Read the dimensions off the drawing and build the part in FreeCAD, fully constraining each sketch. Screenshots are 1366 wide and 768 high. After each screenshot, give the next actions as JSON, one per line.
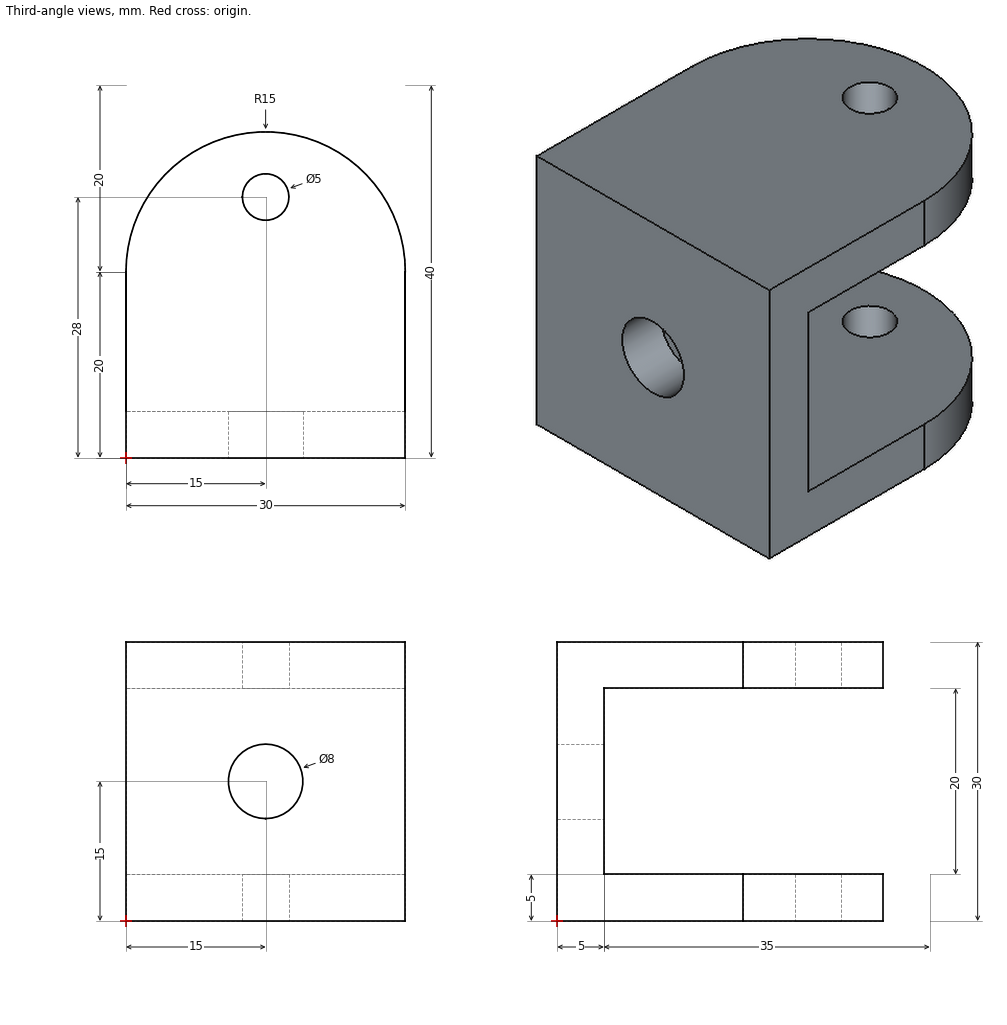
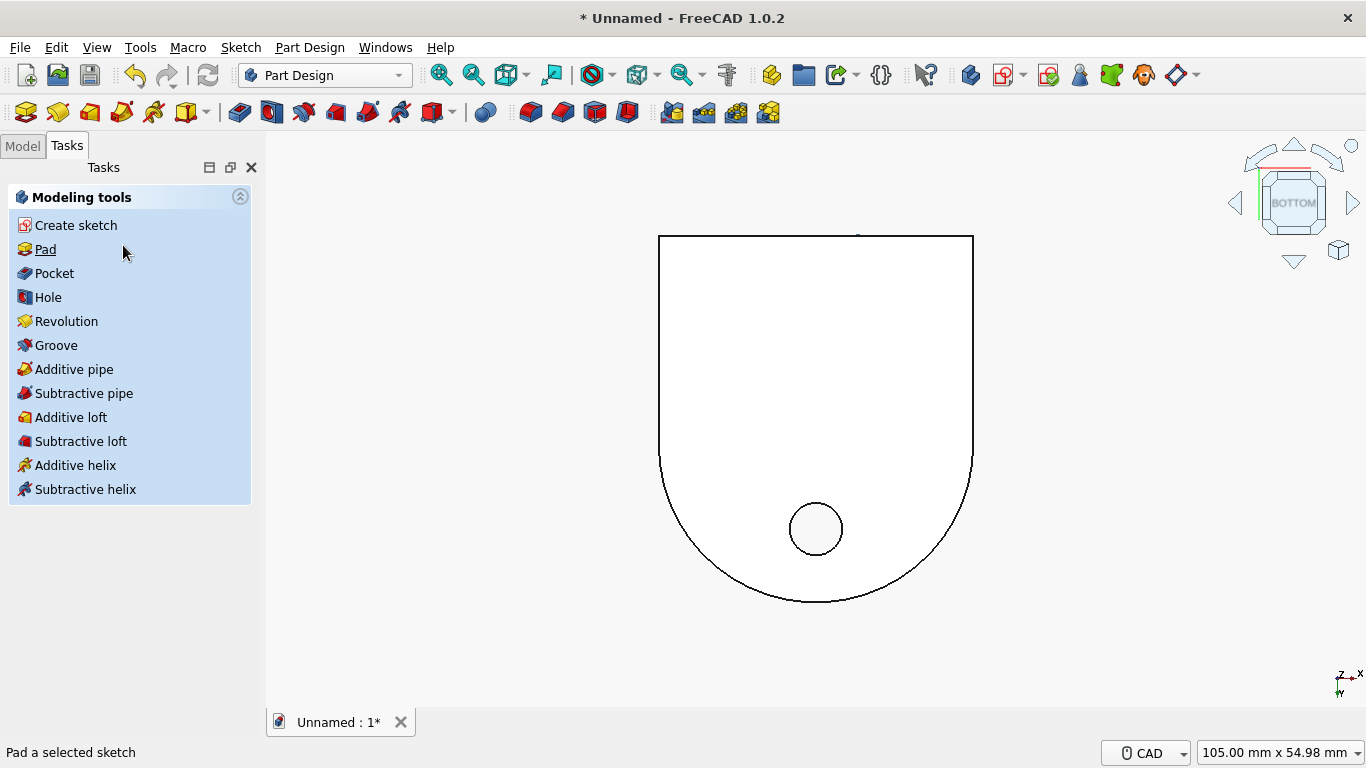
{"action": "left_click", "coordinate": [240, 112]}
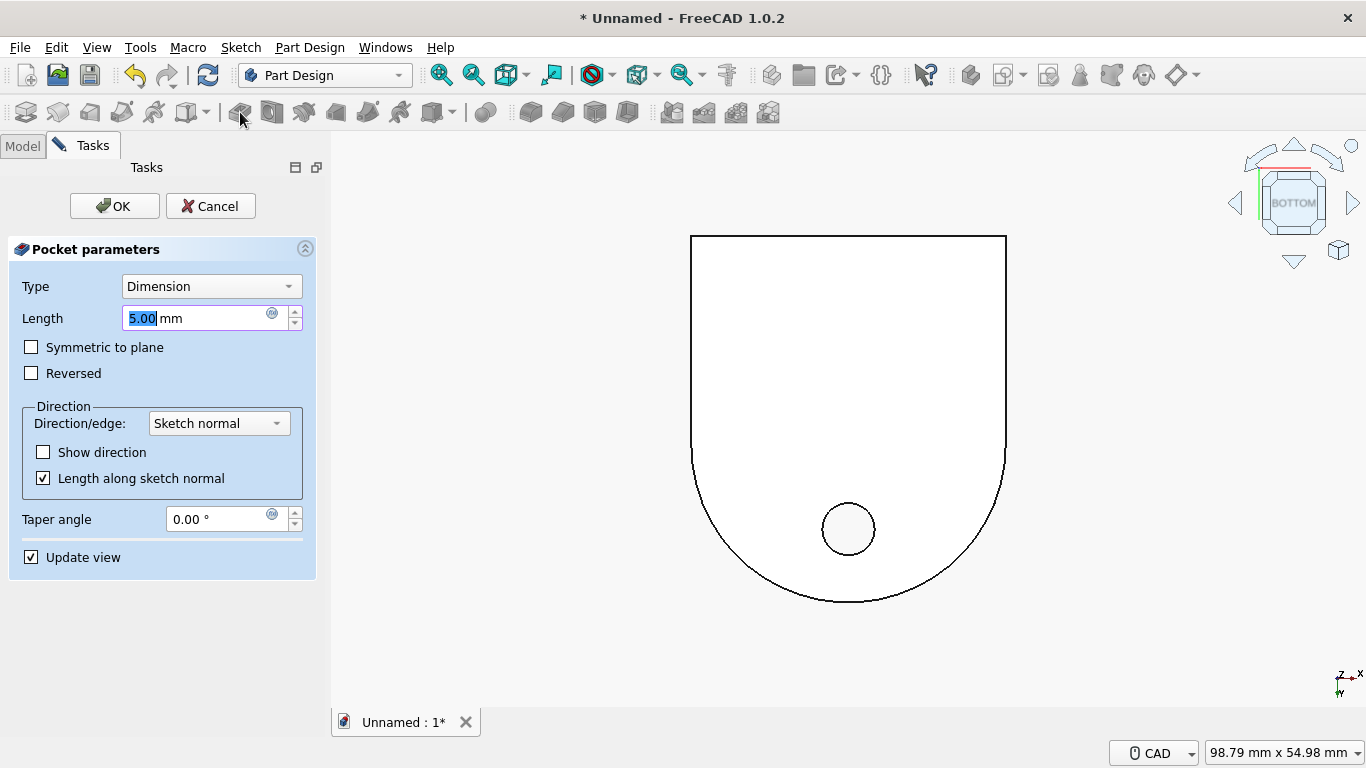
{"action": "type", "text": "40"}
{"action": "key", "text": "Tab"}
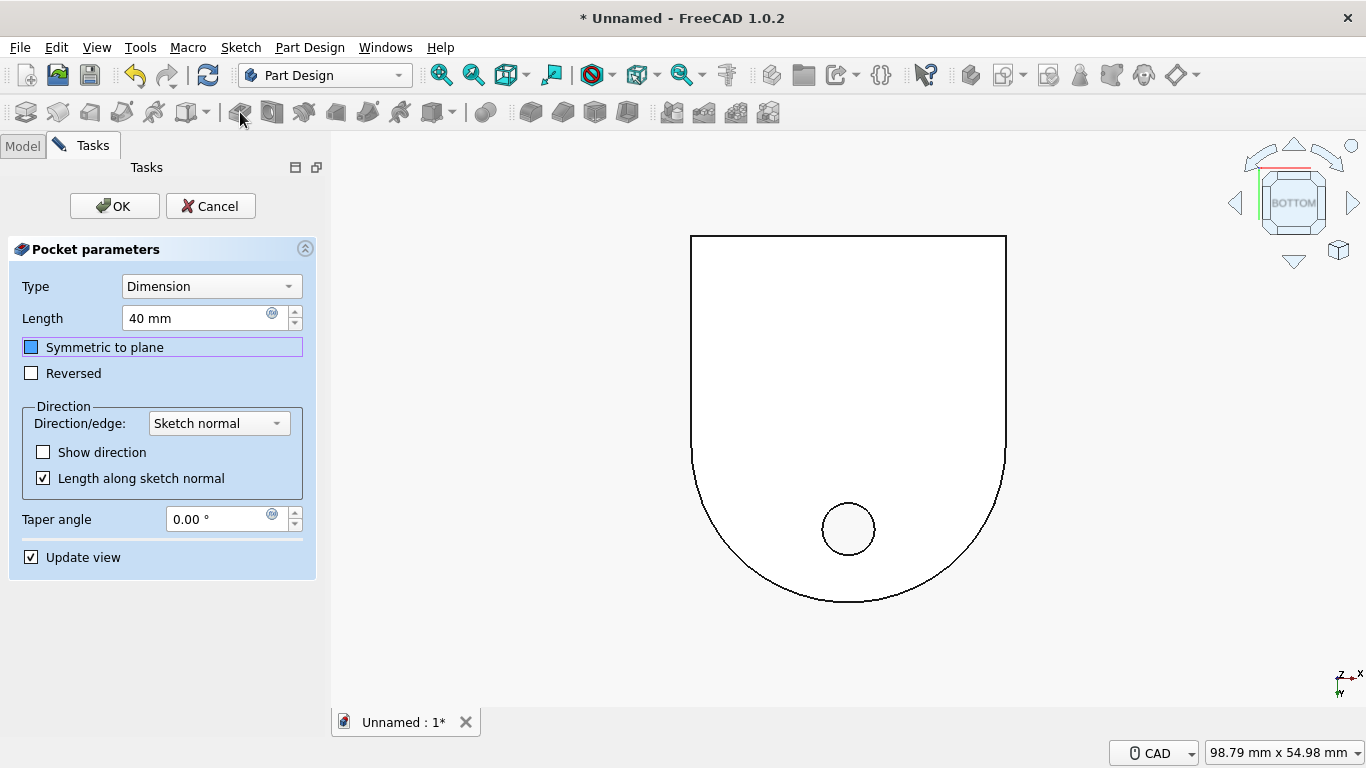
{"action": "left_click", "coordinate": [115, 206]}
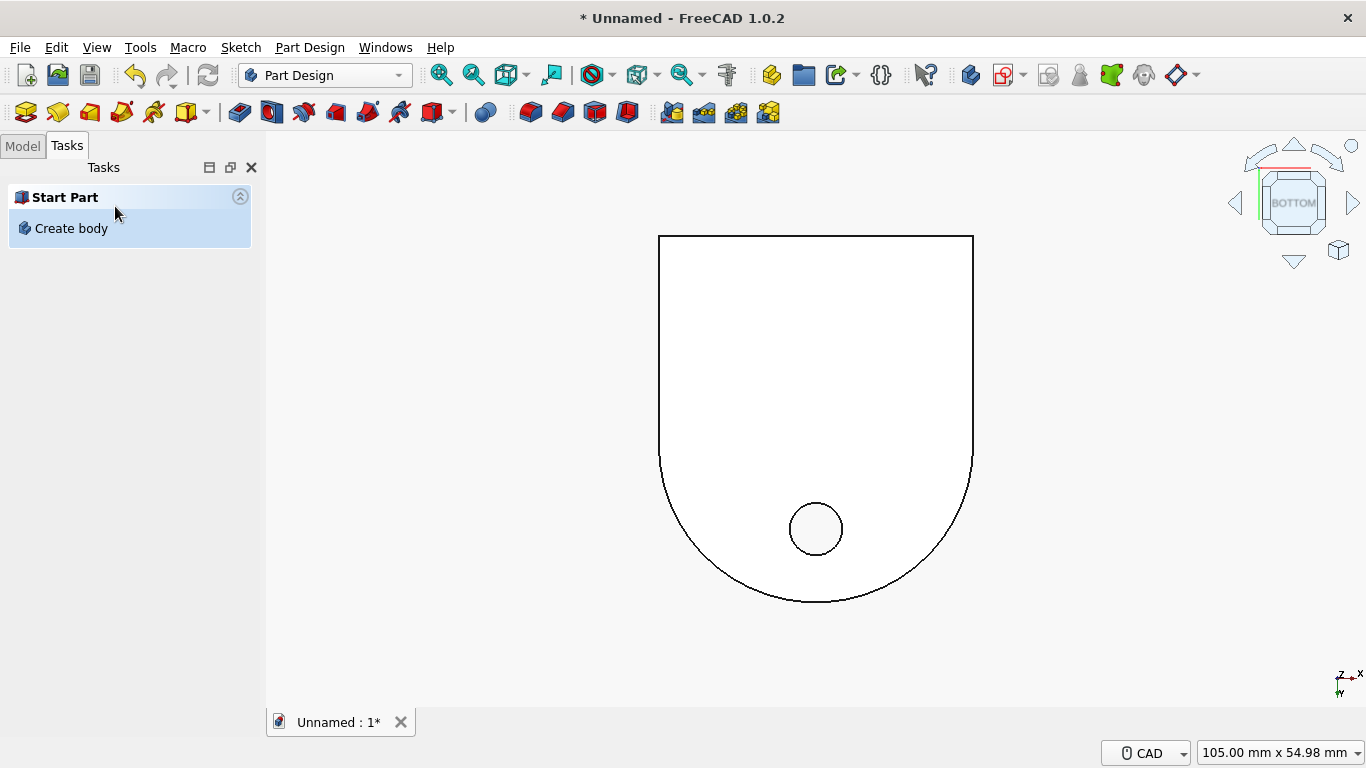
{"action": "key", "text": "0"}